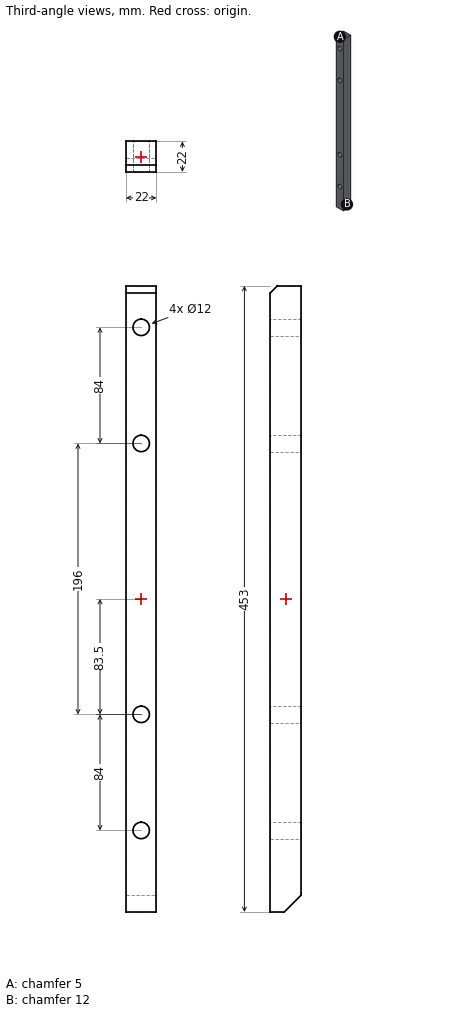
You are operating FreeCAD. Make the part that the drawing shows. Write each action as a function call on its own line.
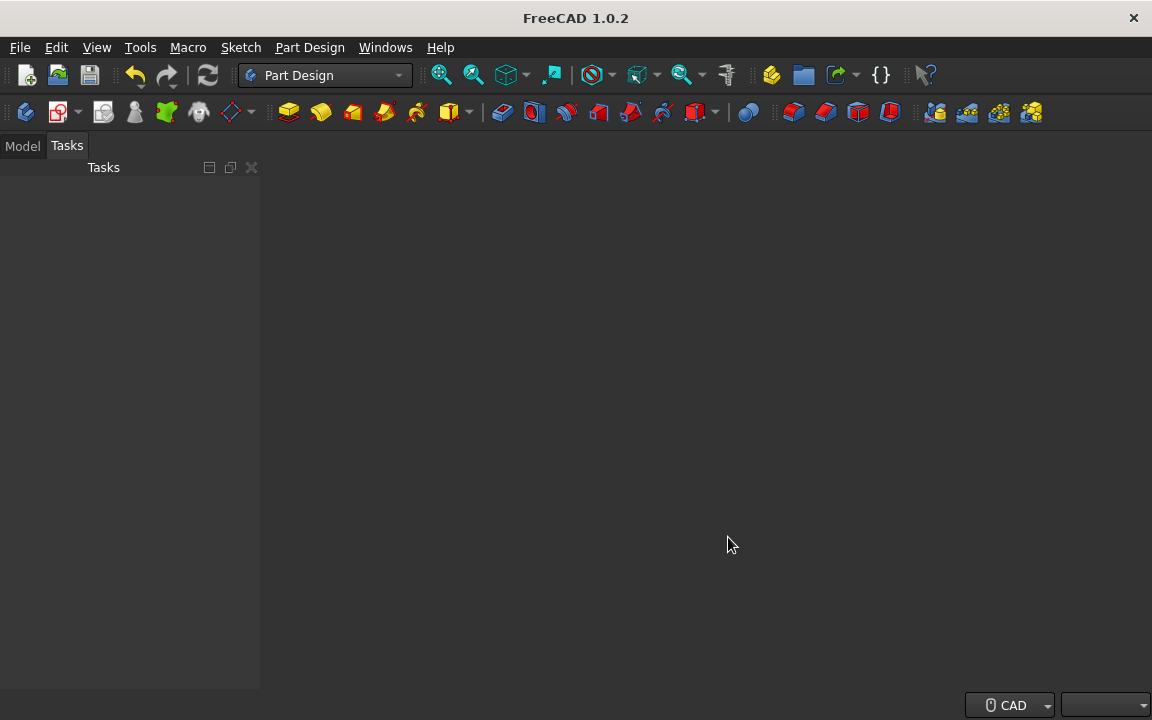
key(ctrl+n)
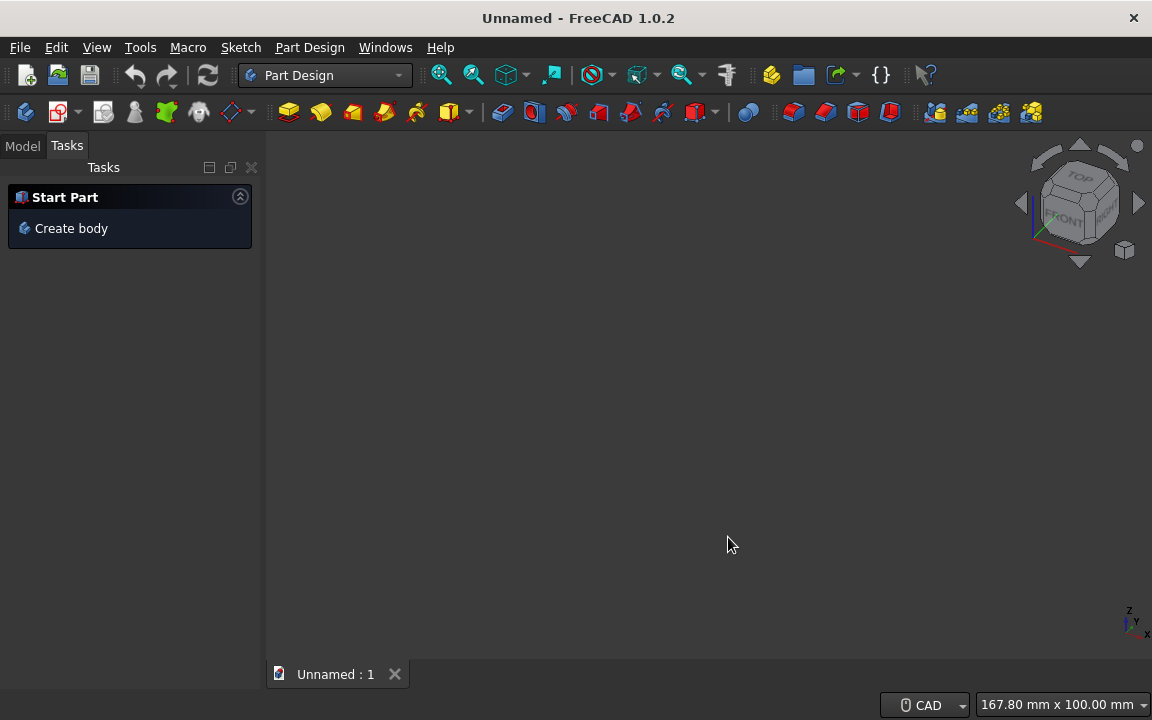
click(58, 112)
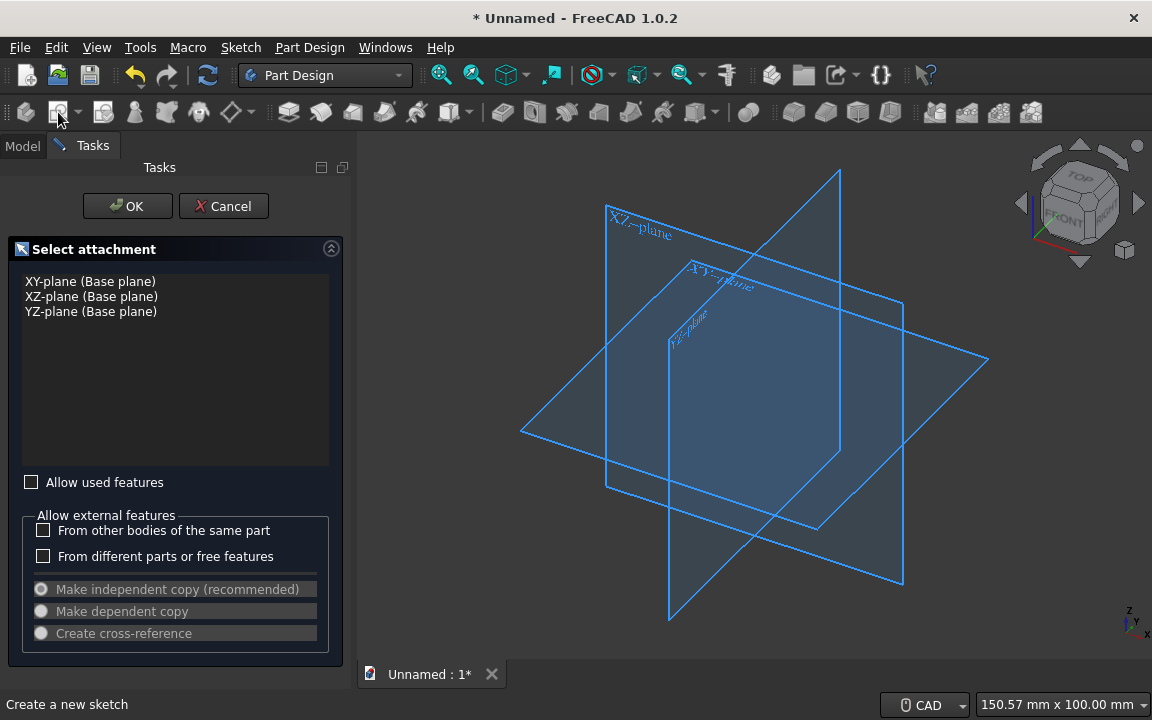
click(82, 282)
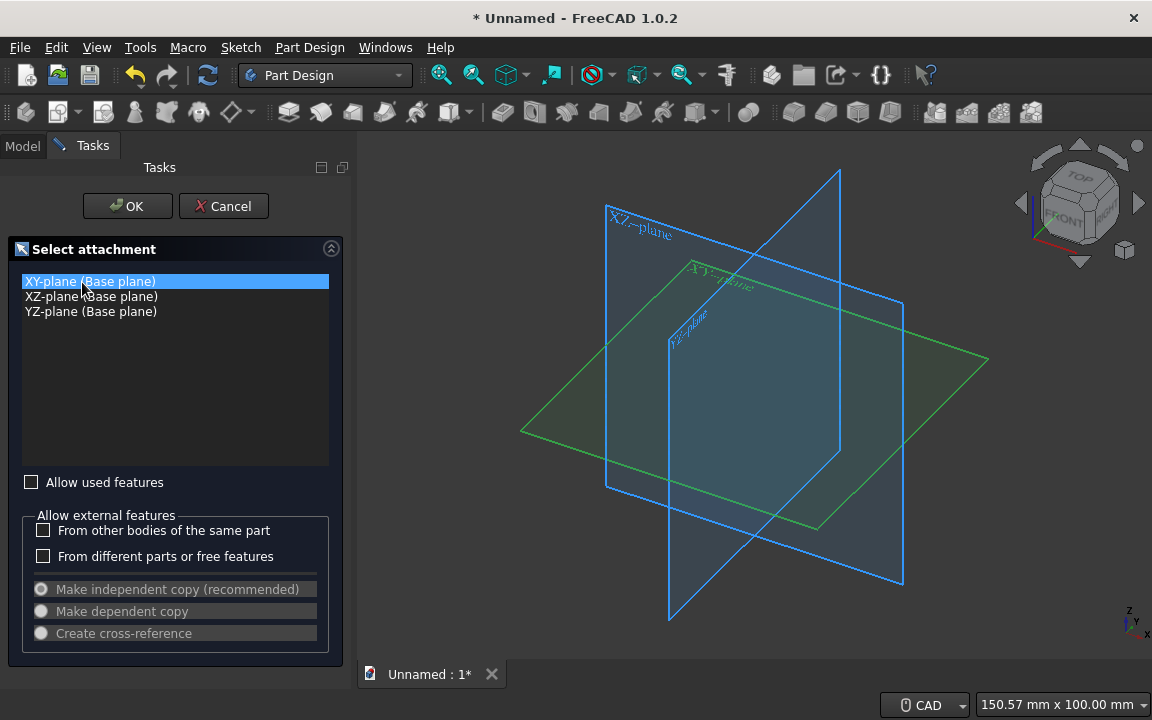
click(128, 206)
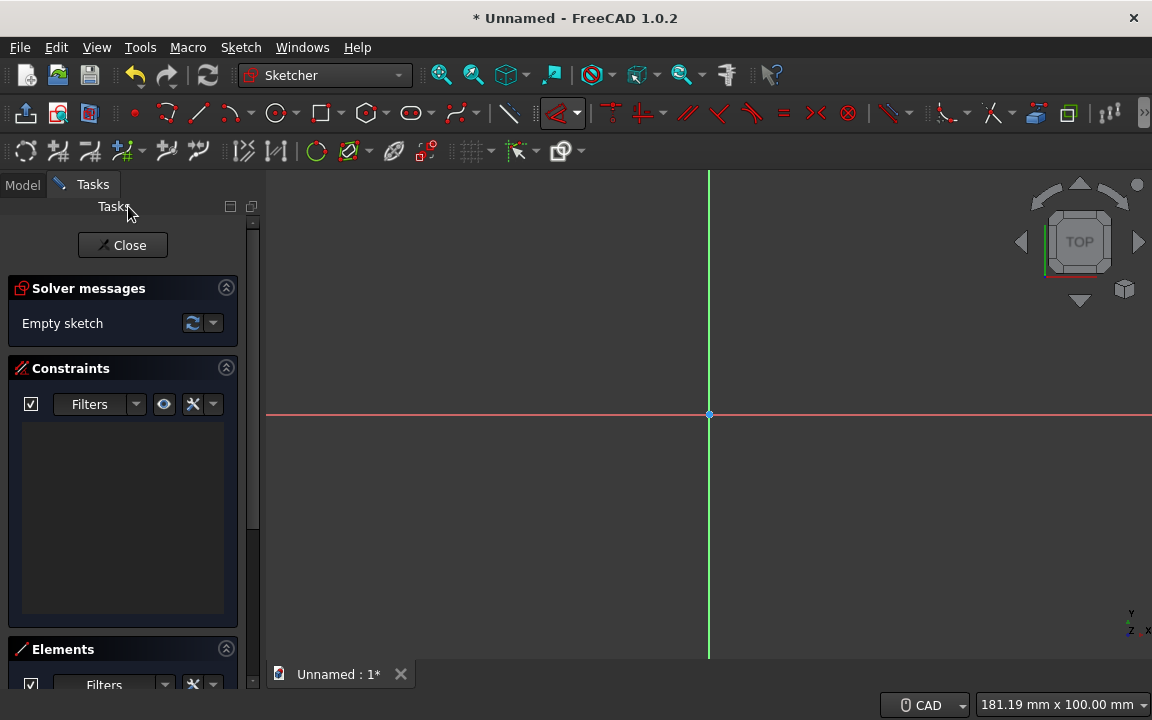
scroll(749, 415, up, 5)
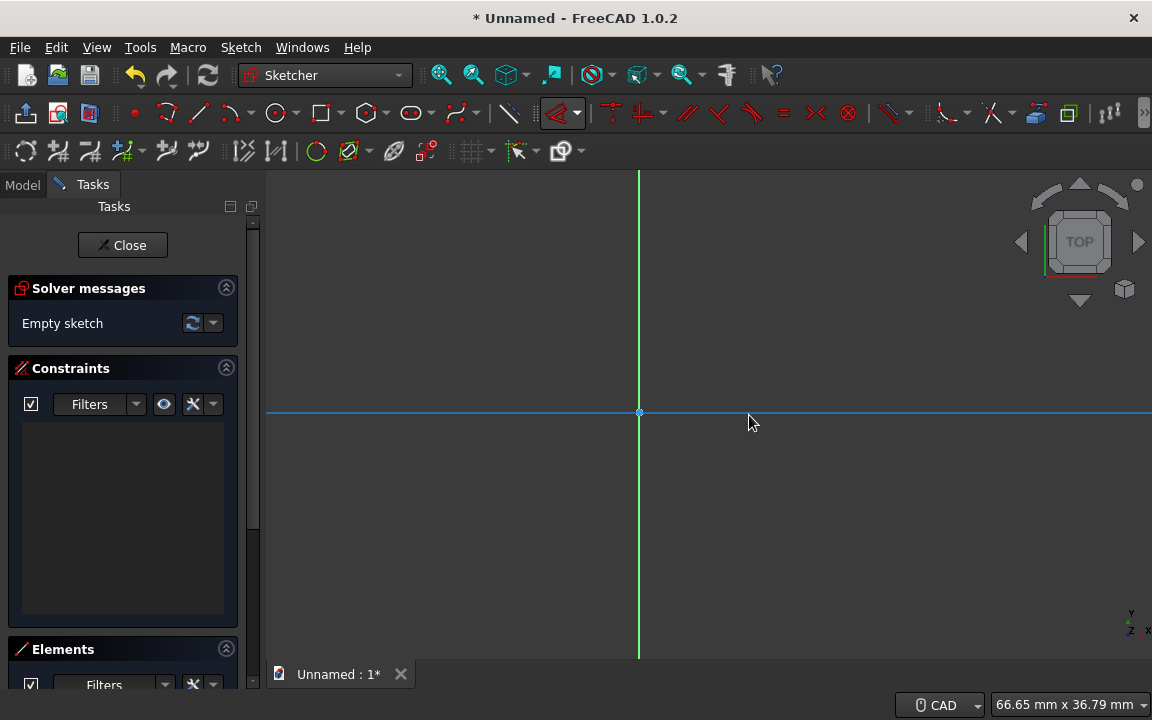
key(g)
key(v)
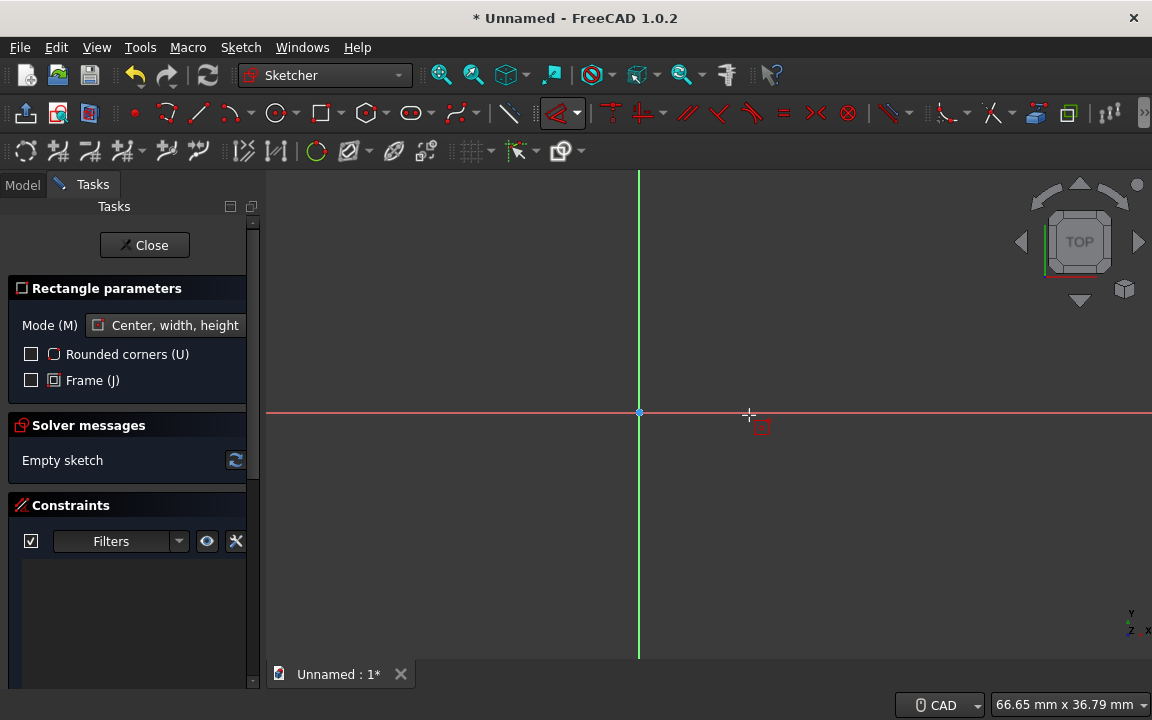
click(639, 413)
move(786, 267)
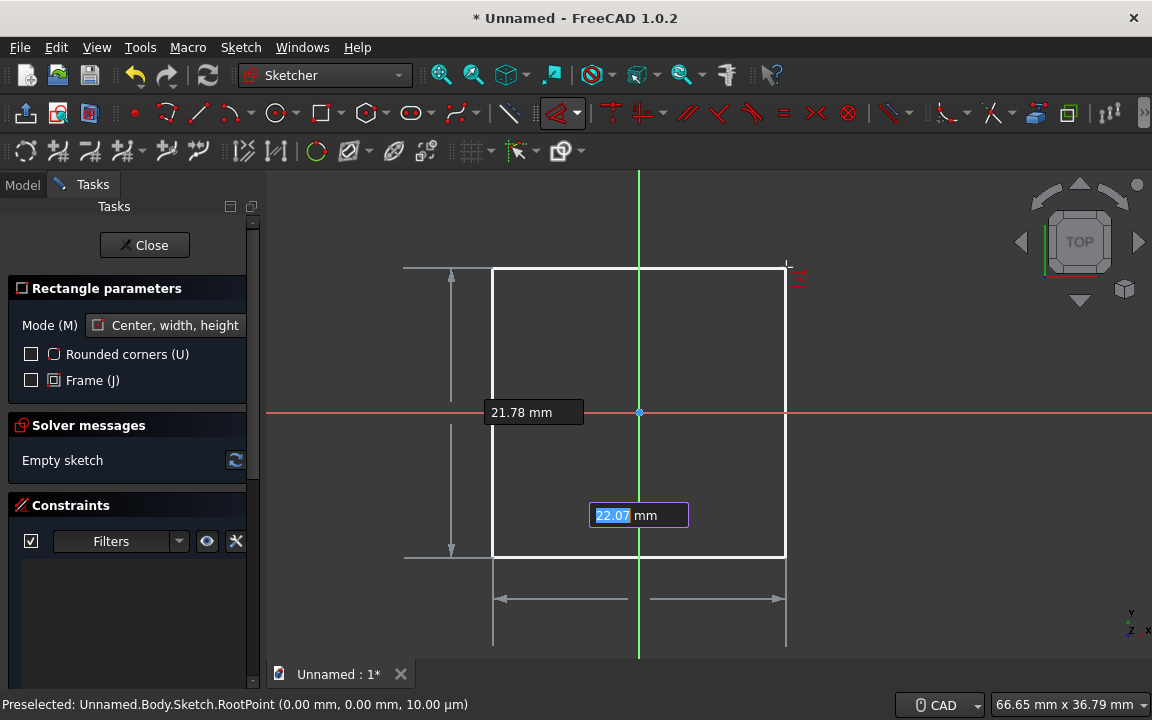
text(22)
key(Tab)
text(22)
key(Return)
key(Escape)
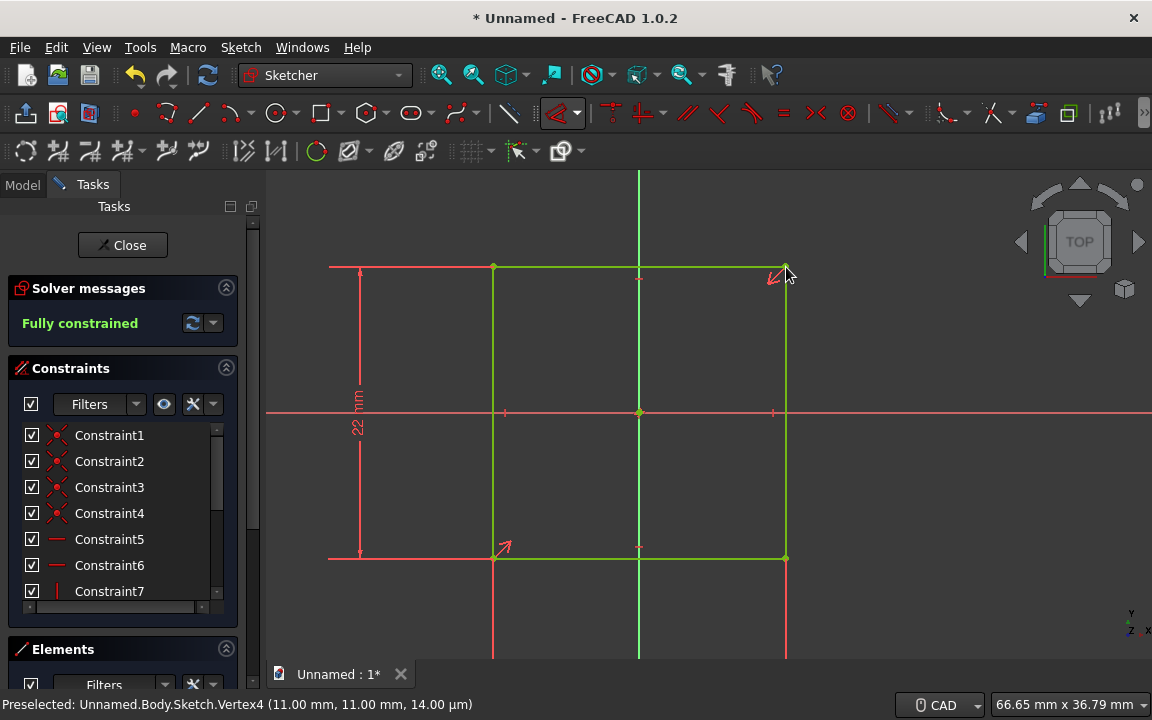
click(123, 245)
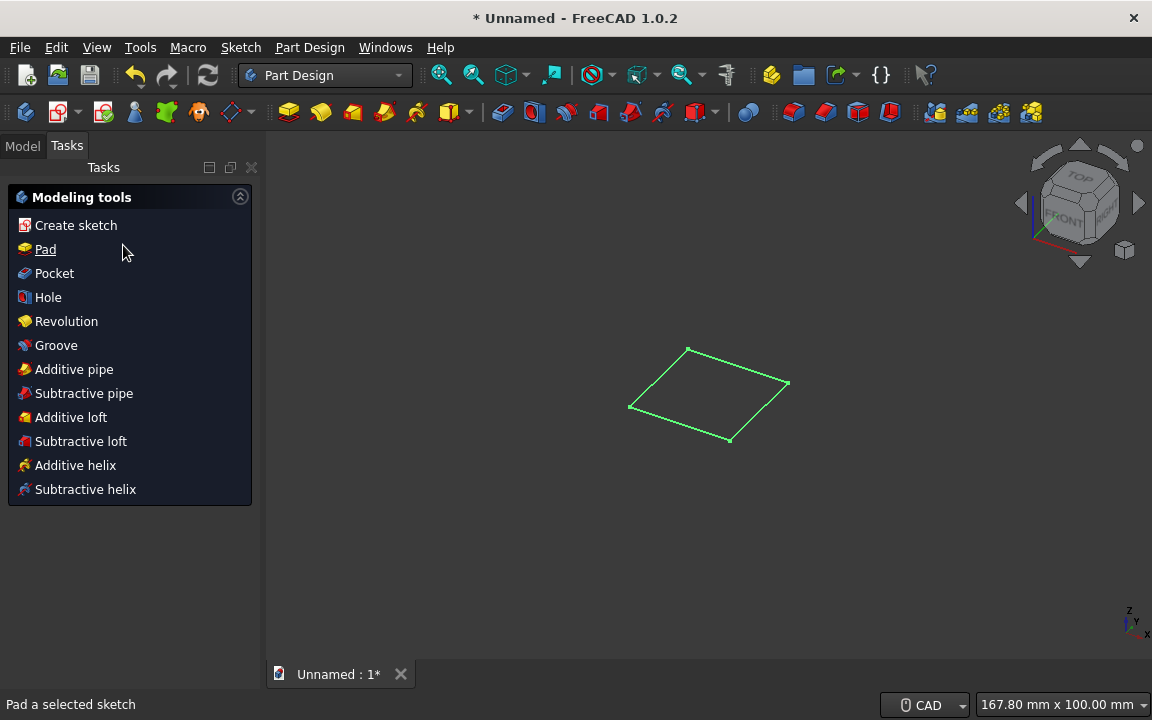
click(290, 112)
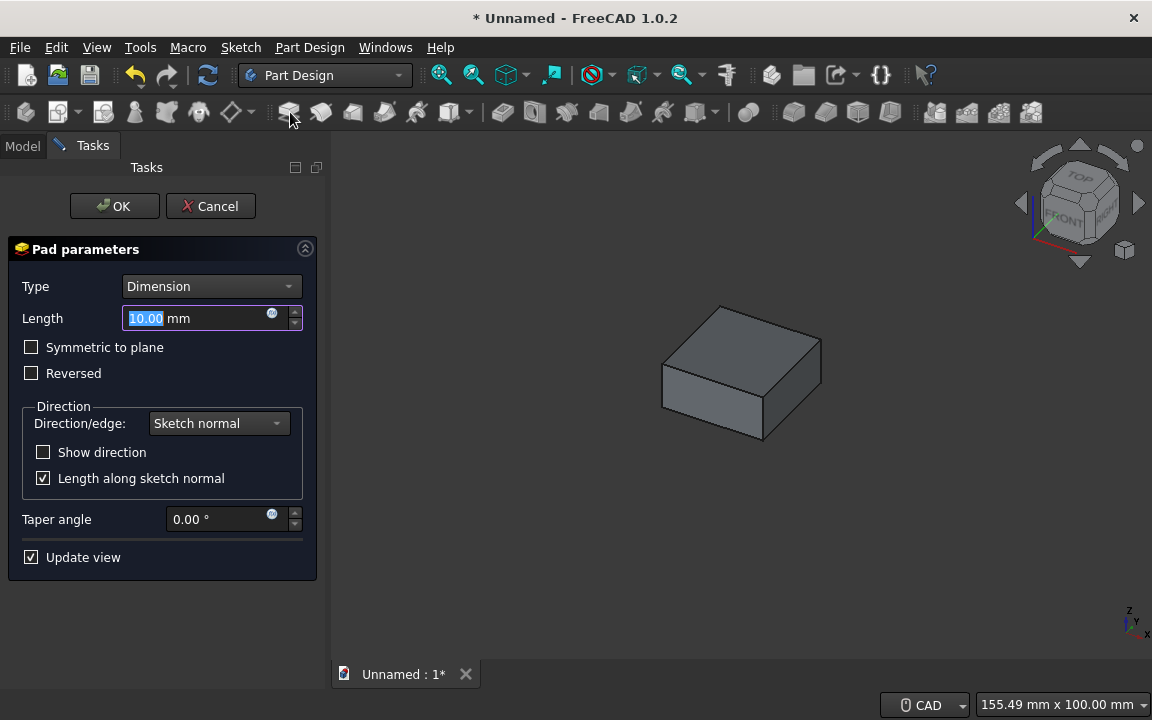
text(453)
key(Tab)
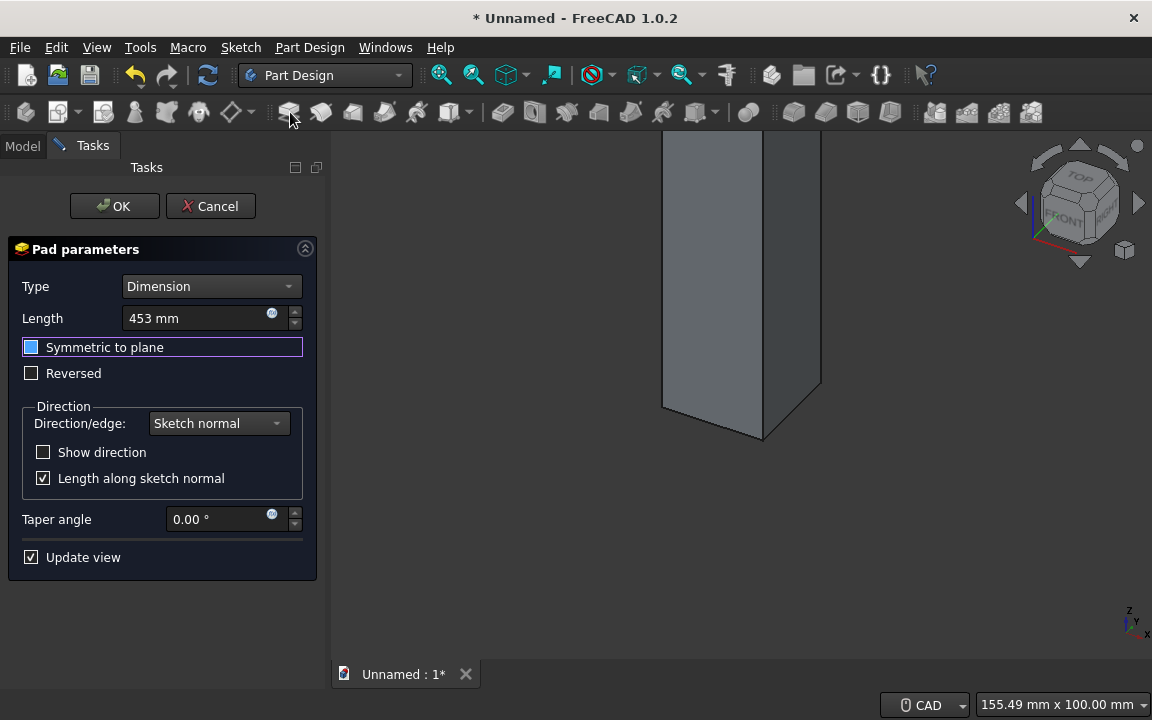
click(30, 347)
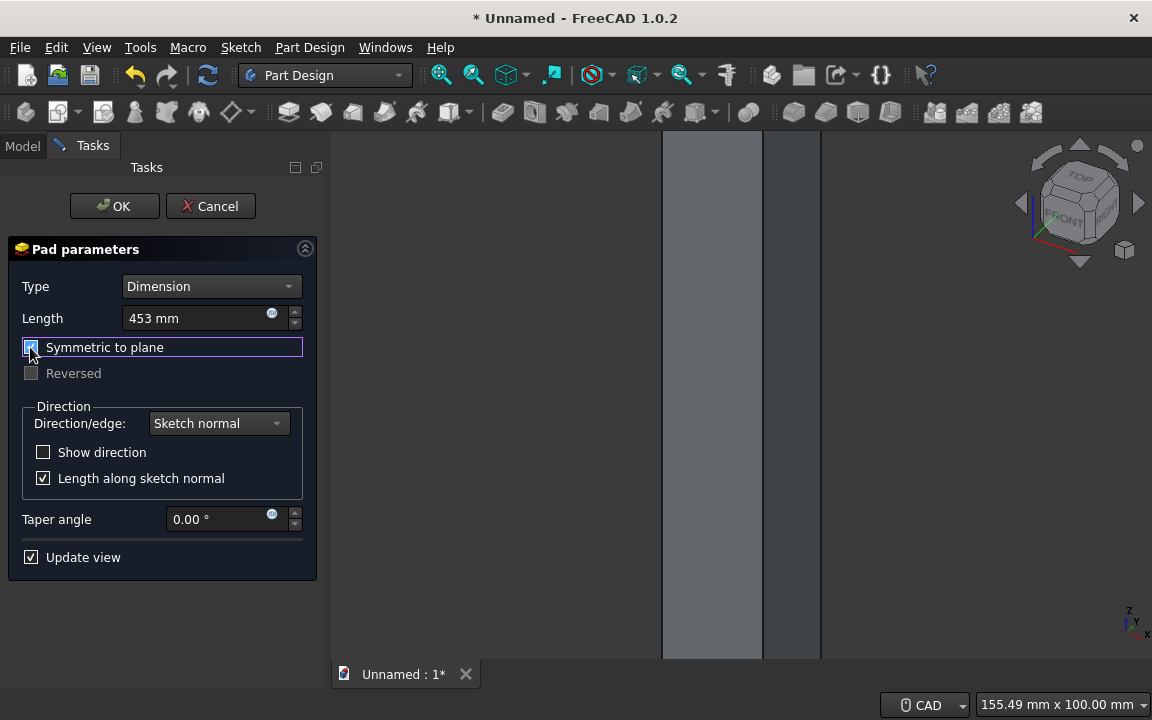
click(115, 206)